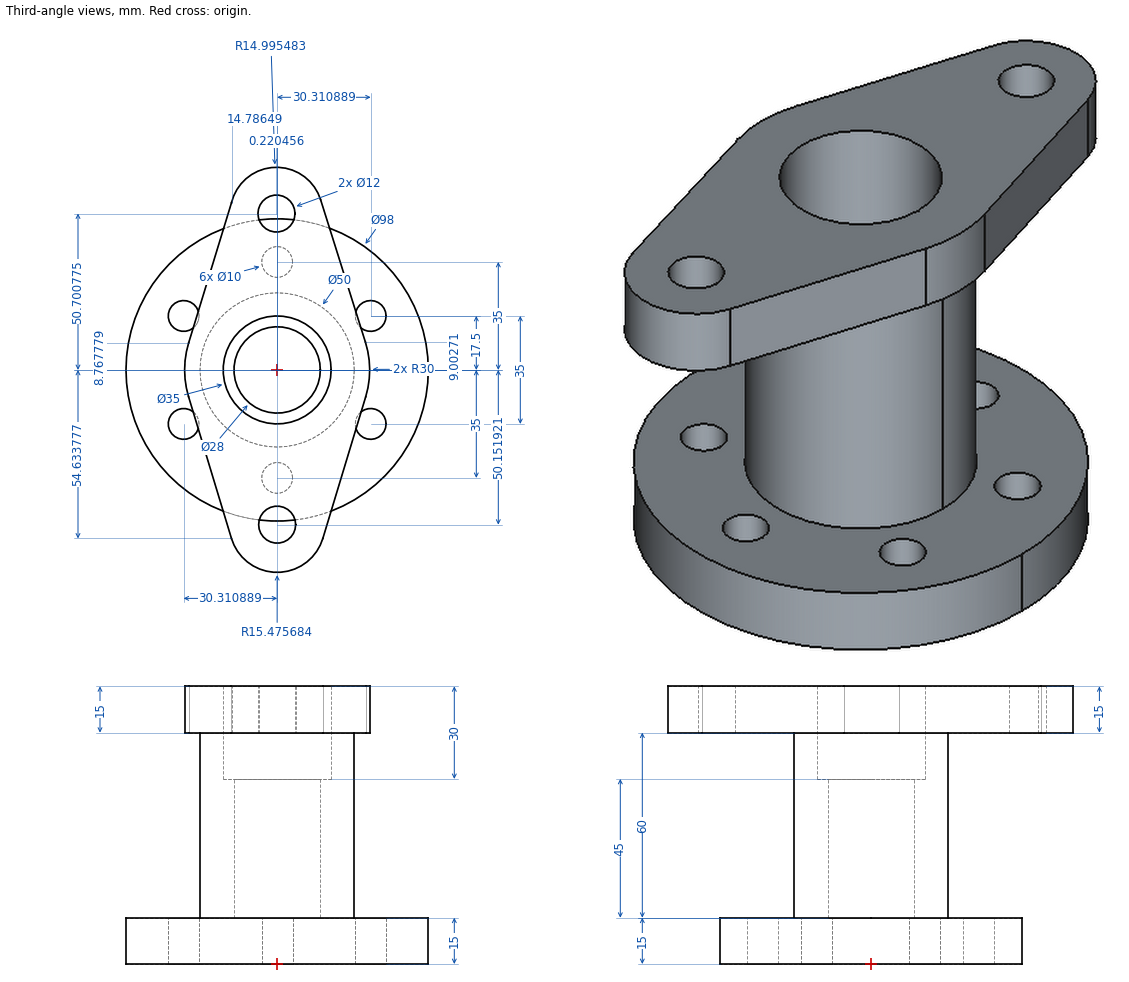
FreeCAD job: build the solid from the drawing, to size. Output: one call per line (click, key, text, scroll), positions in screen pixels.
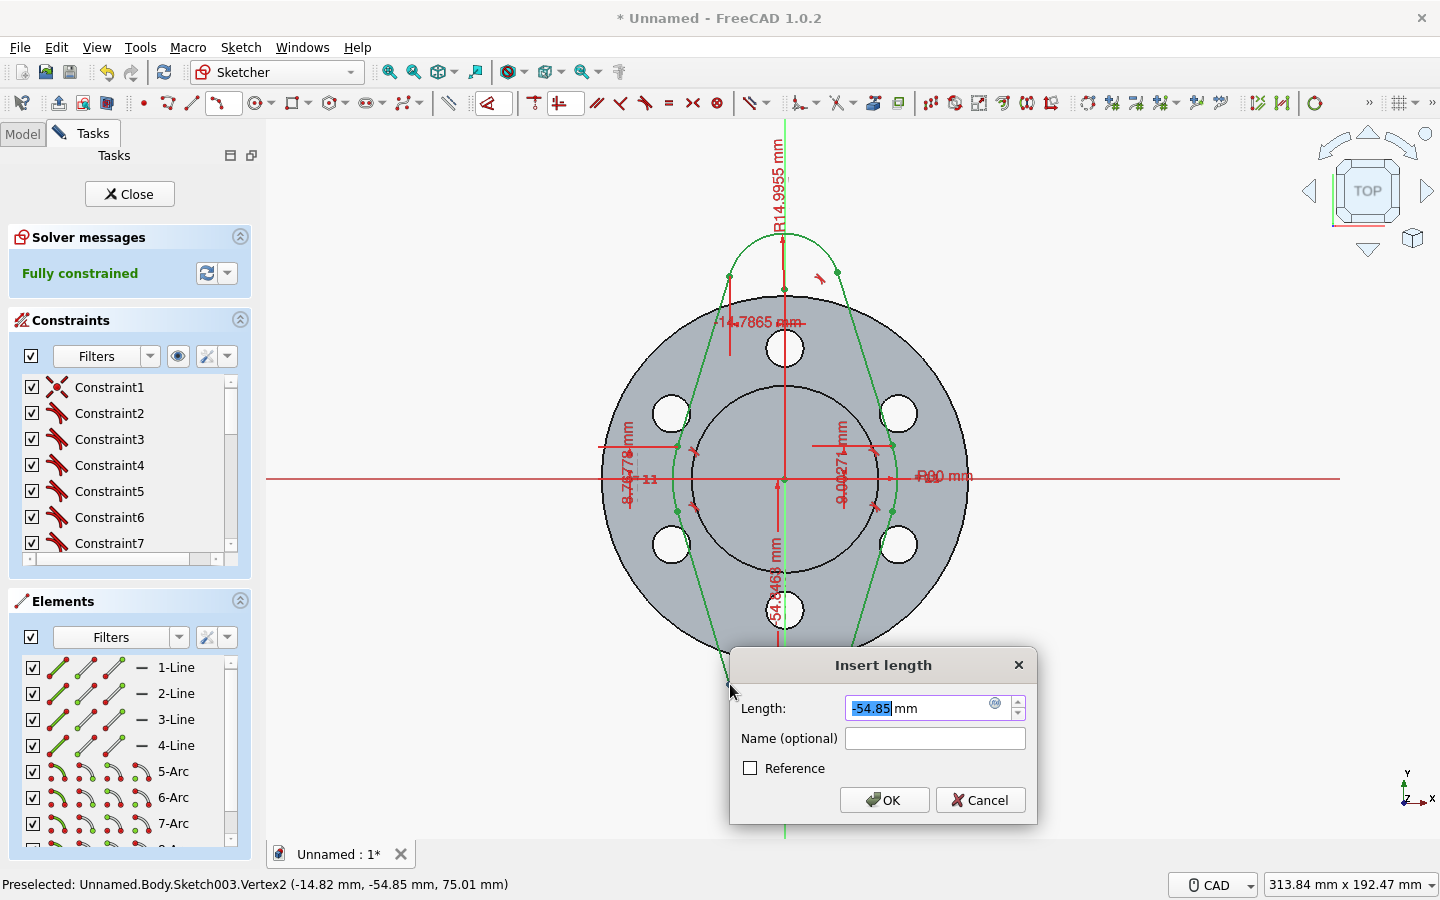
text(-54.633777)
key(Return)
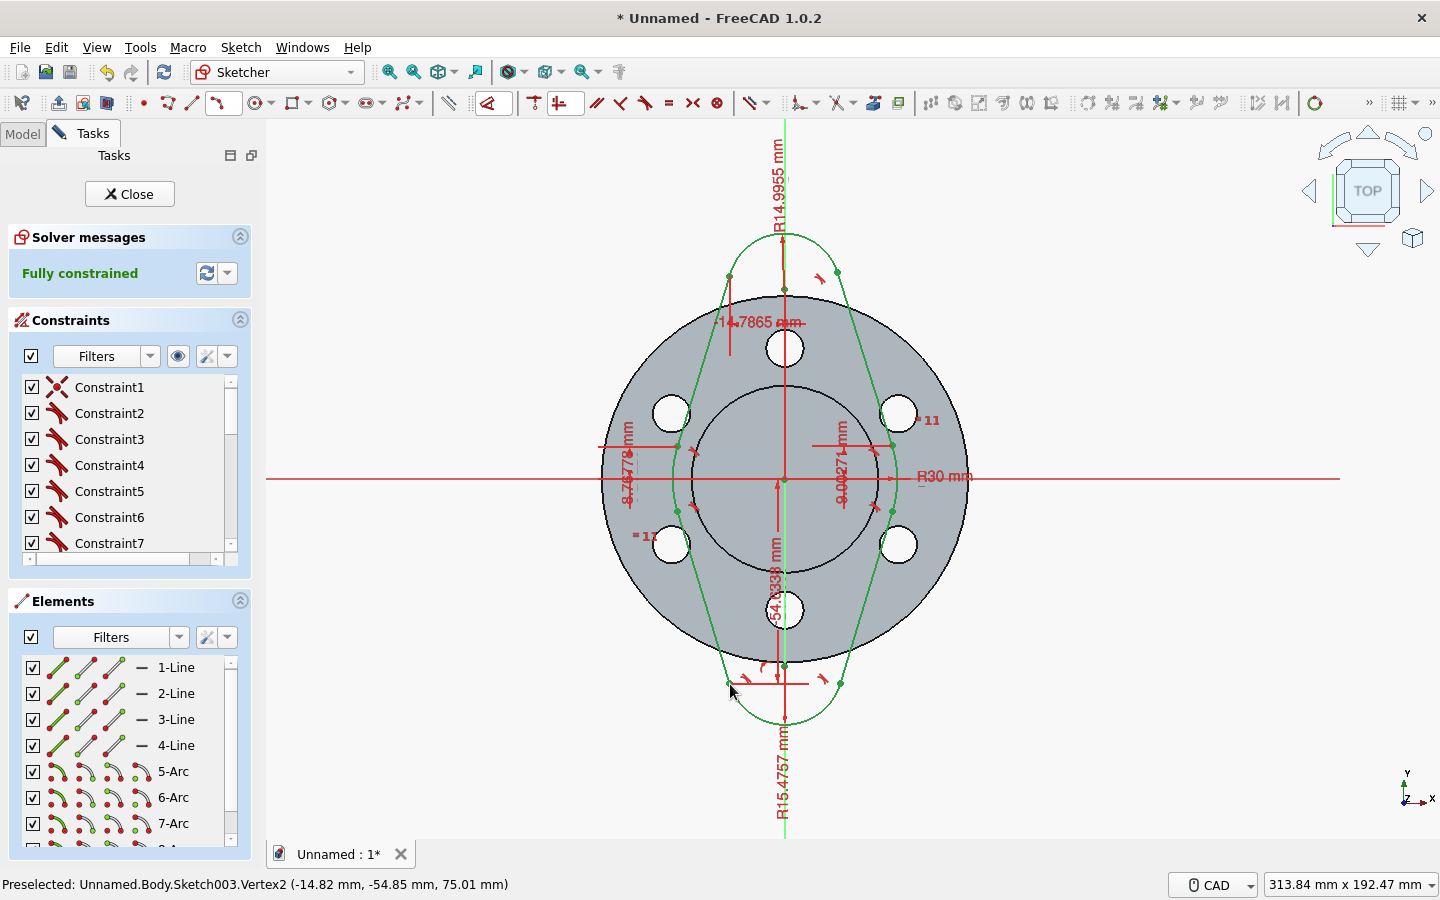
click(130, 194)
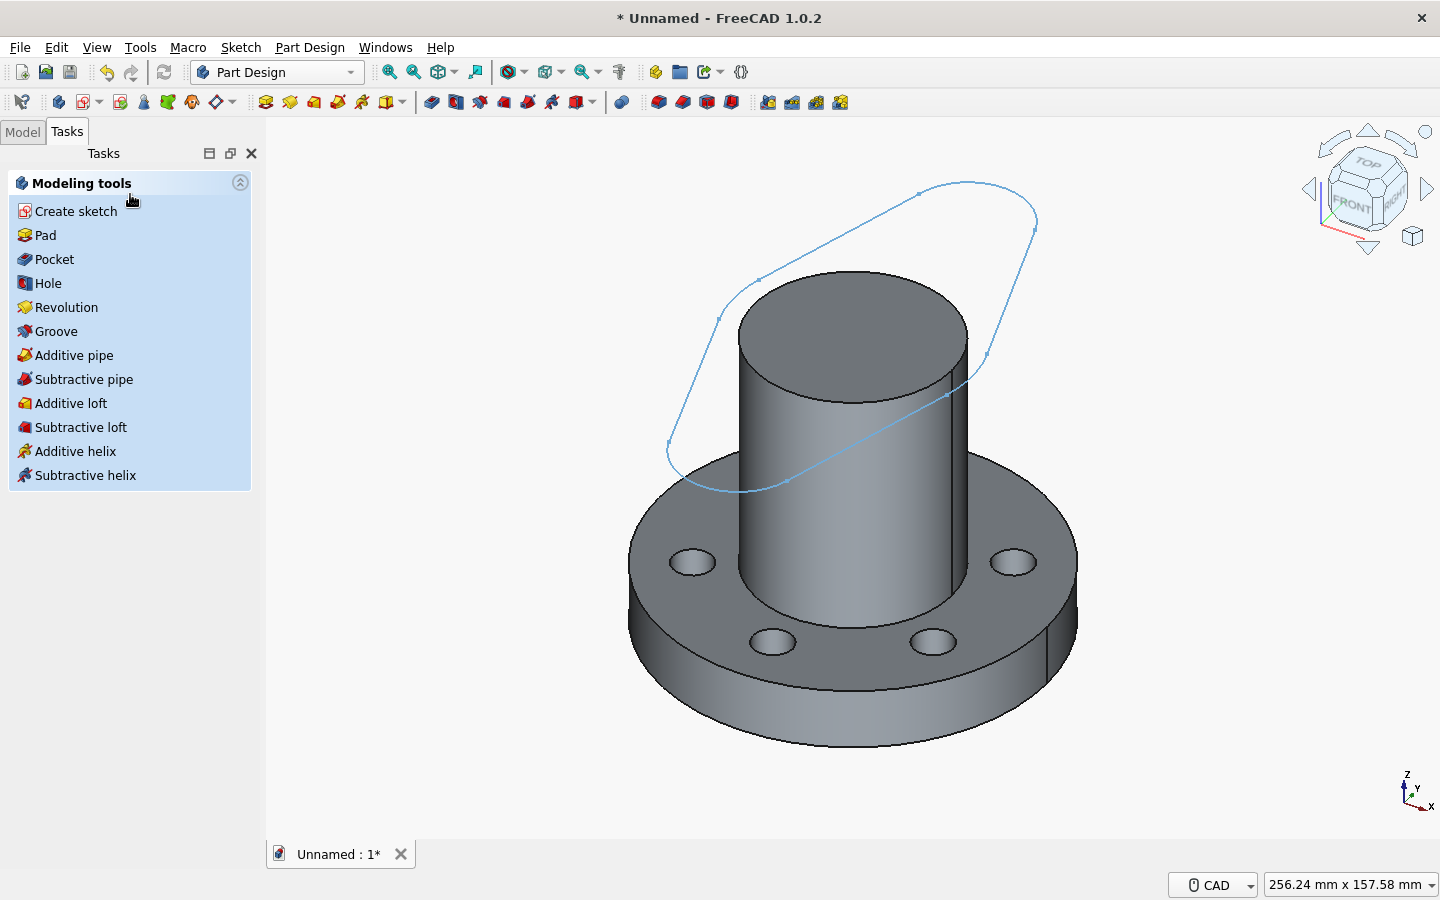
click(266, 102)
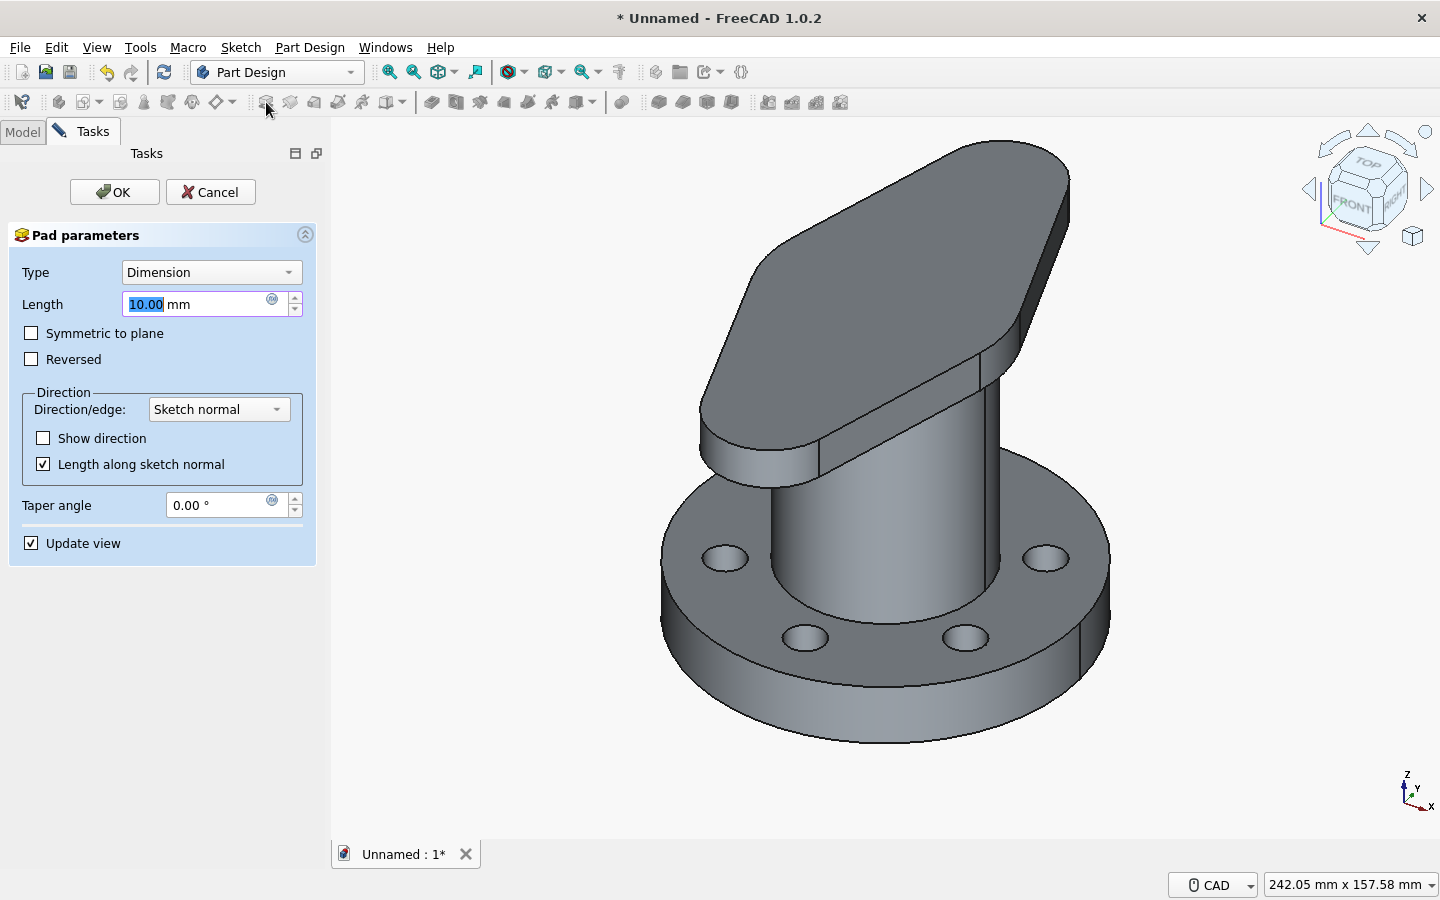
text(15)
key(Tab)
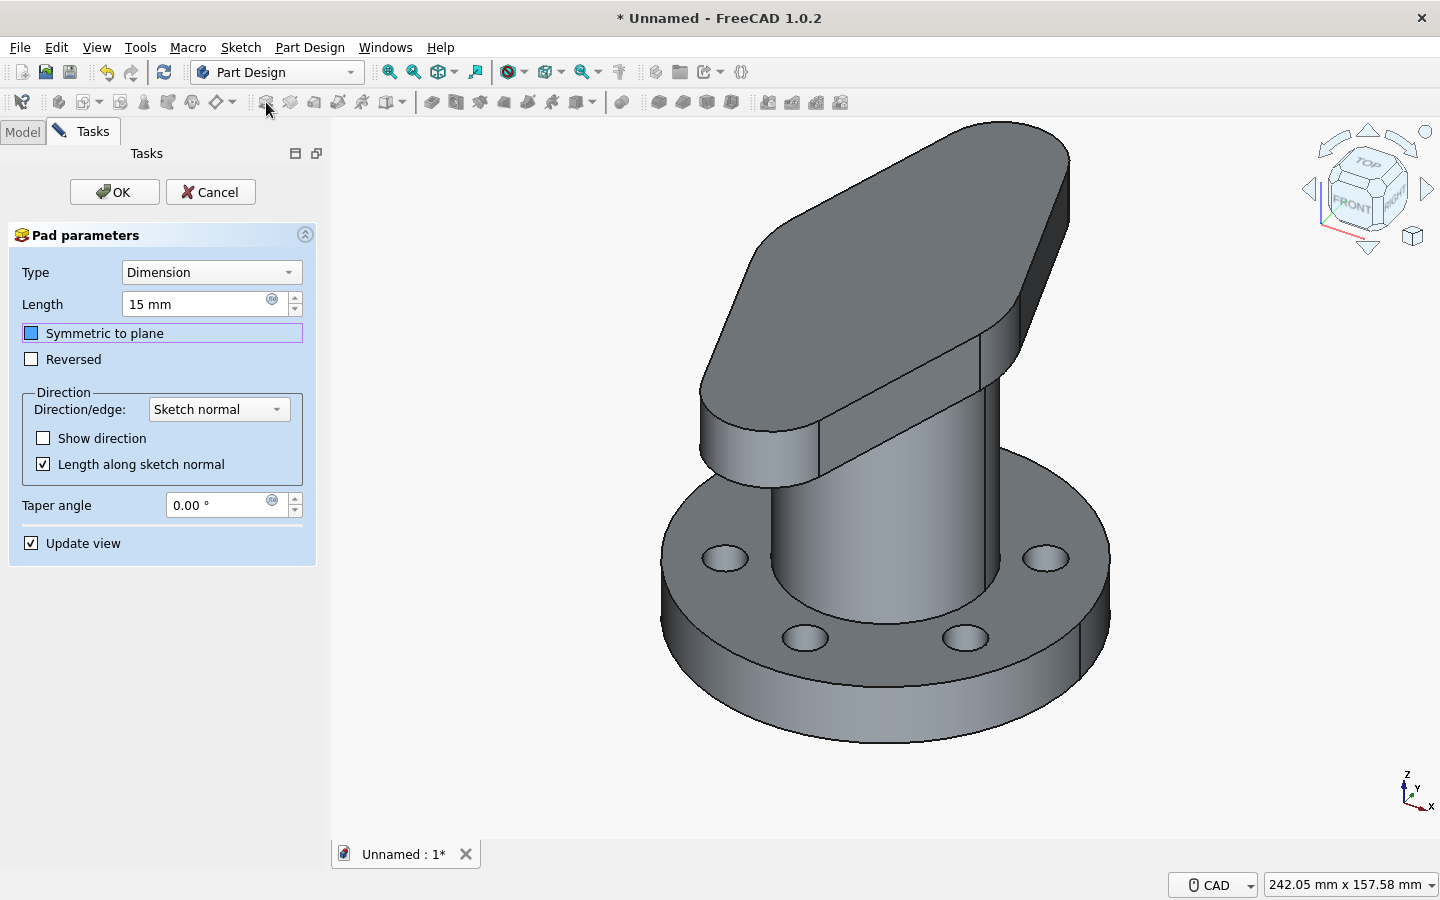
click(115, 192)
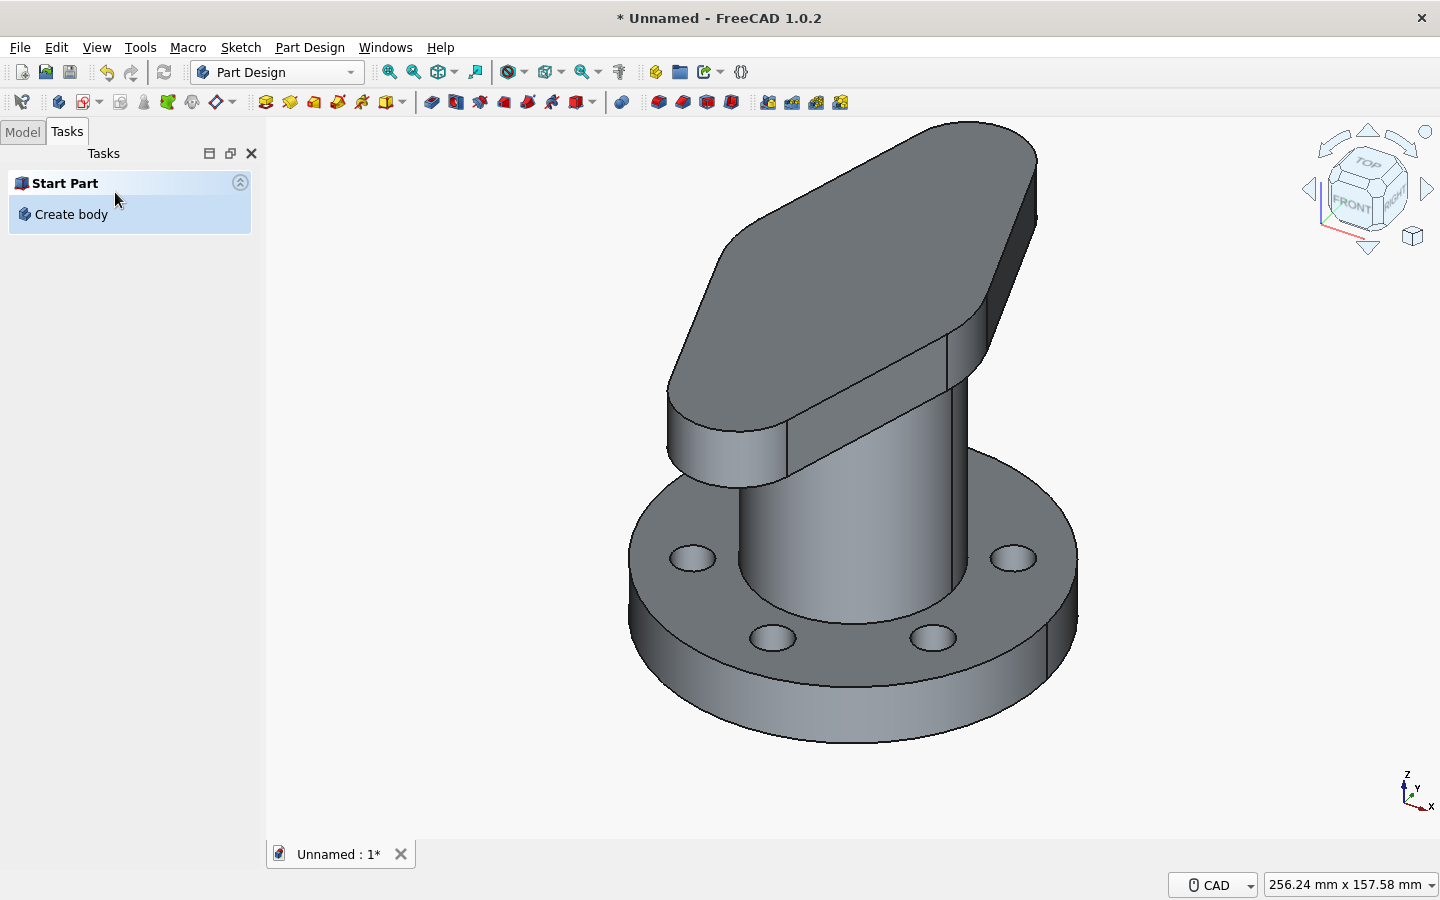
key(v)
key(f)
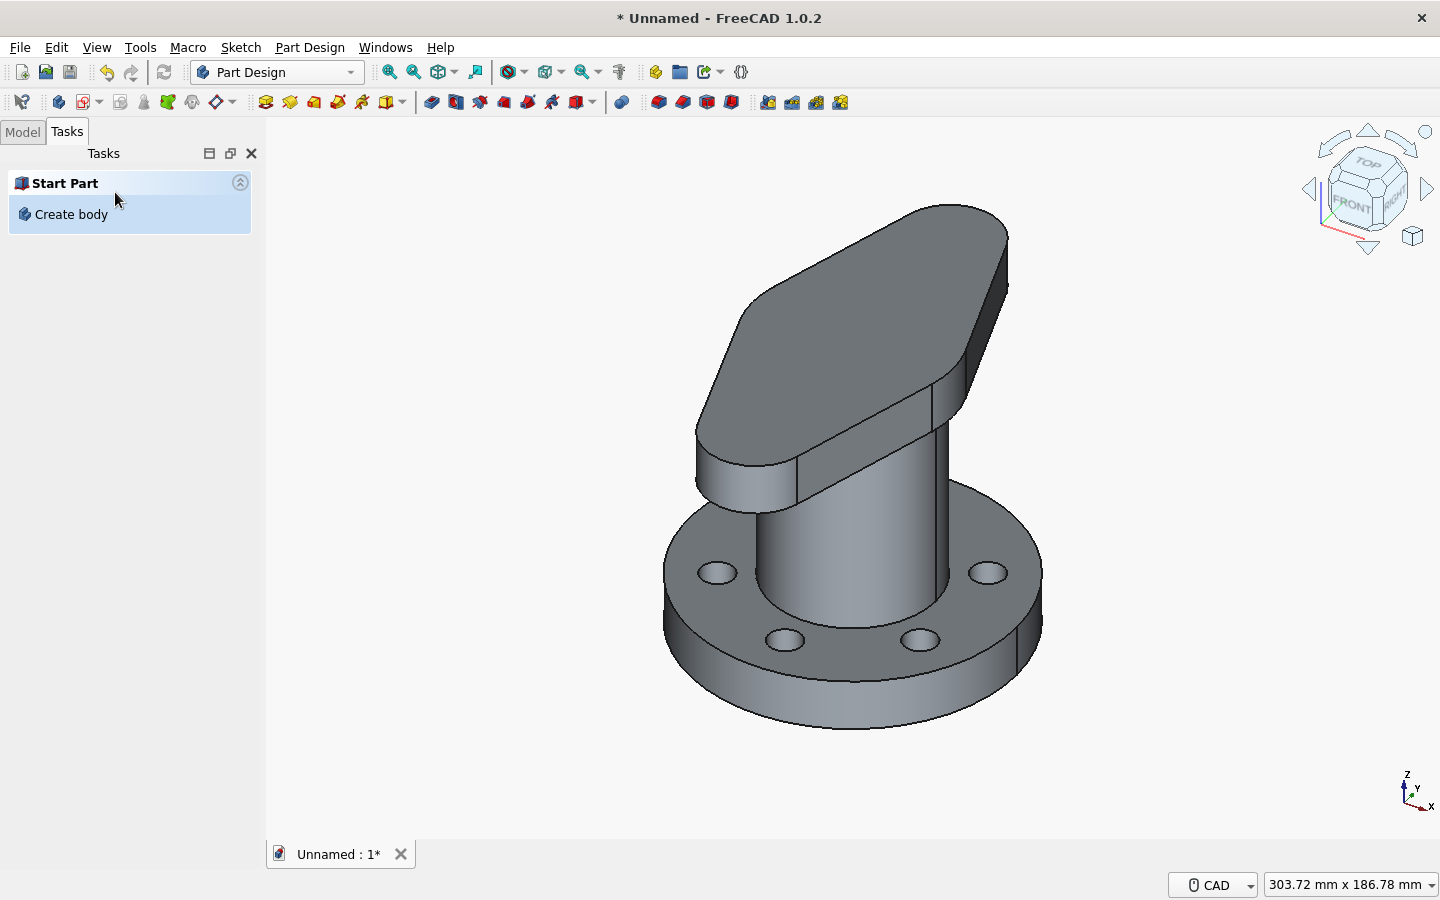
click(853, 335)